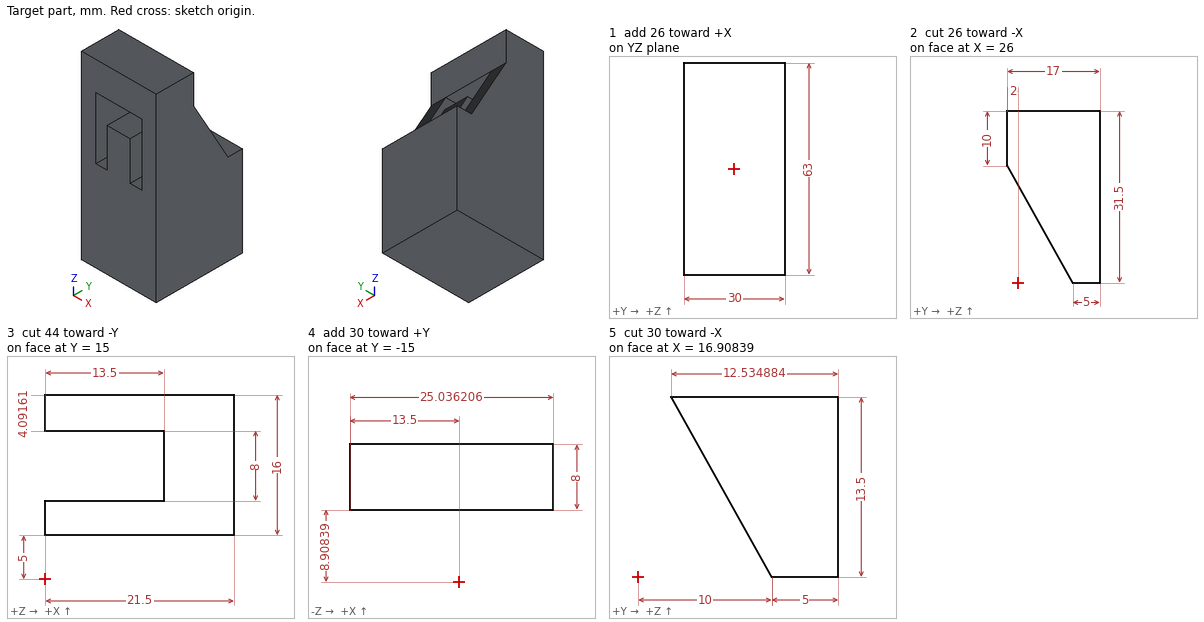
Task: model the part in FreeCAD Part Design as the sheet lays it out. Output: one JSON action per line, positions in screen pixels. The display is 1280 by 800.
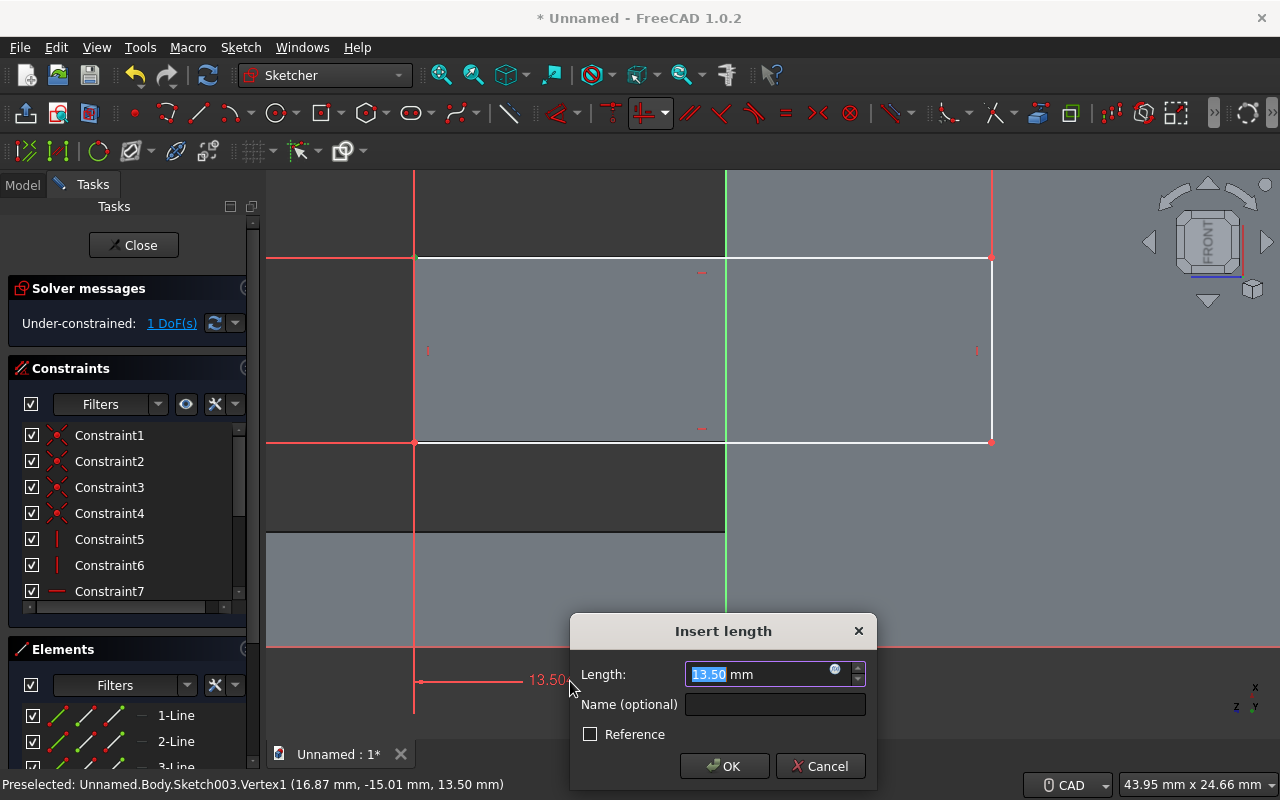
{"action": "type", "text": "13.5"}
{"action": "key", "text": "Return"}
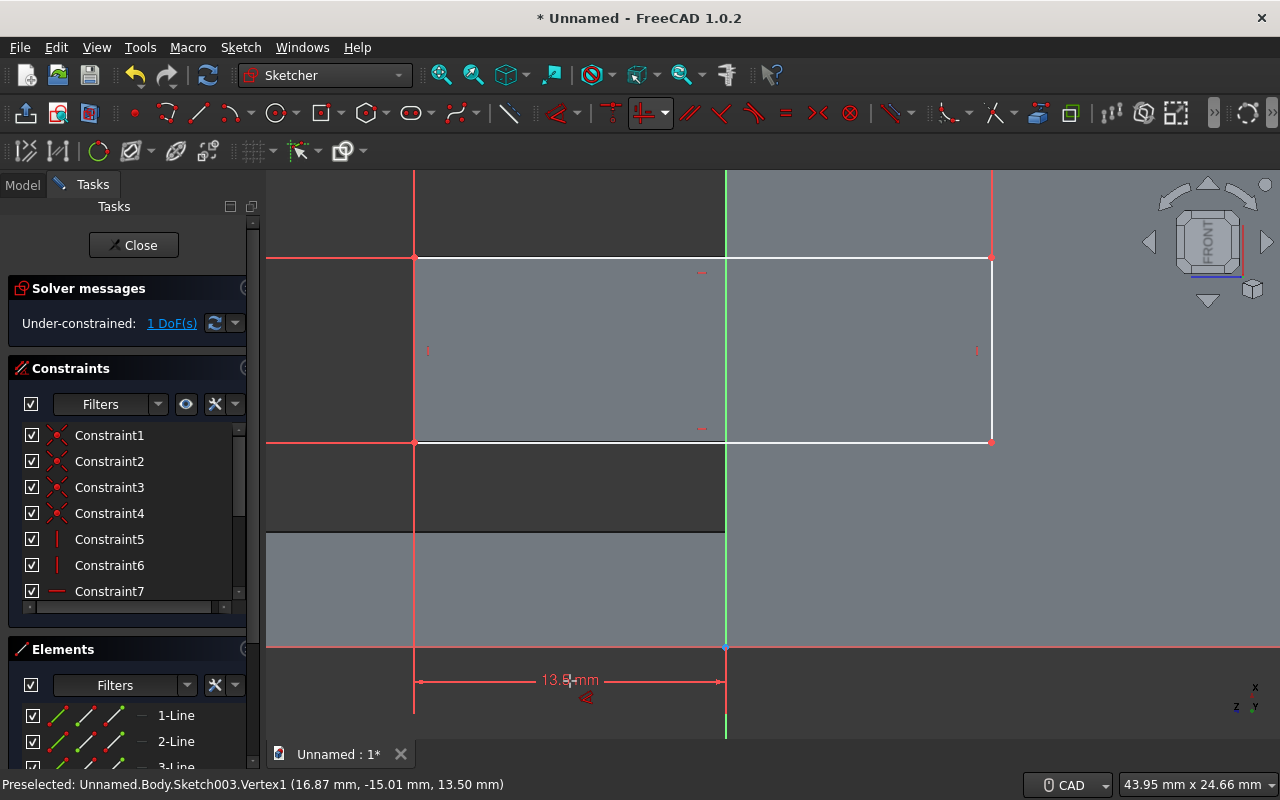
{"action": "left_click", "coordinate": [414, 443]}
{"action": "left_click", "coordinate": [380, 545]}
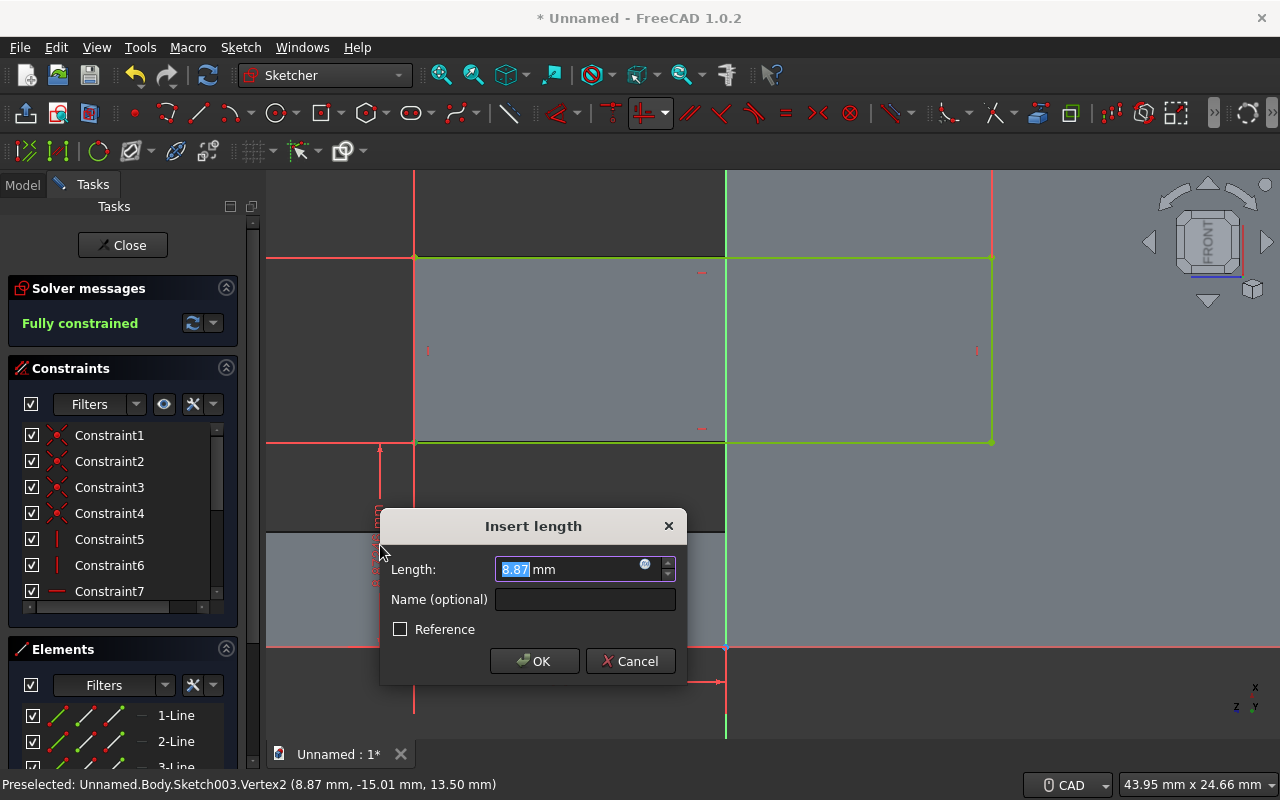
{"action": "type", "text": "8.90839"}
{"action": "key", "text": "Return"}
{"action": "key", "text": "Escape"}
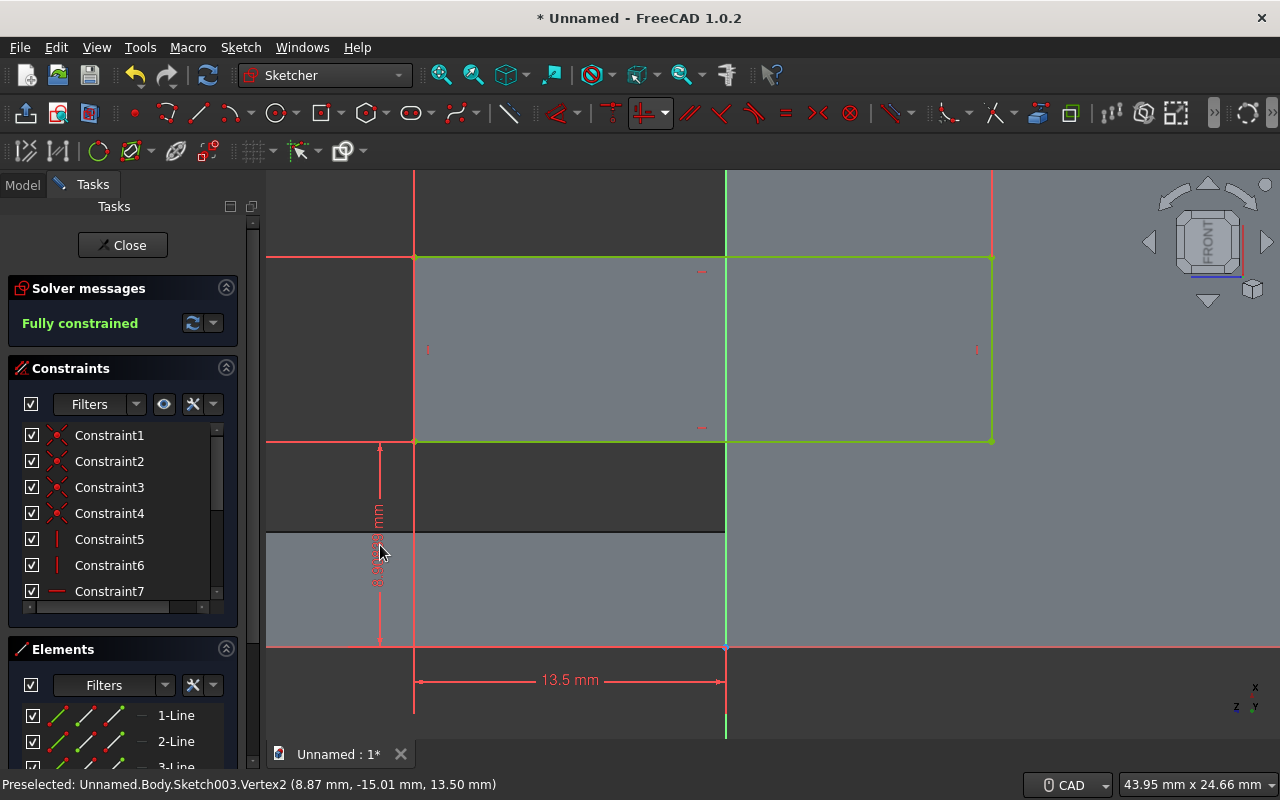
{"action": "left_click", "coordinate": [123, 245]}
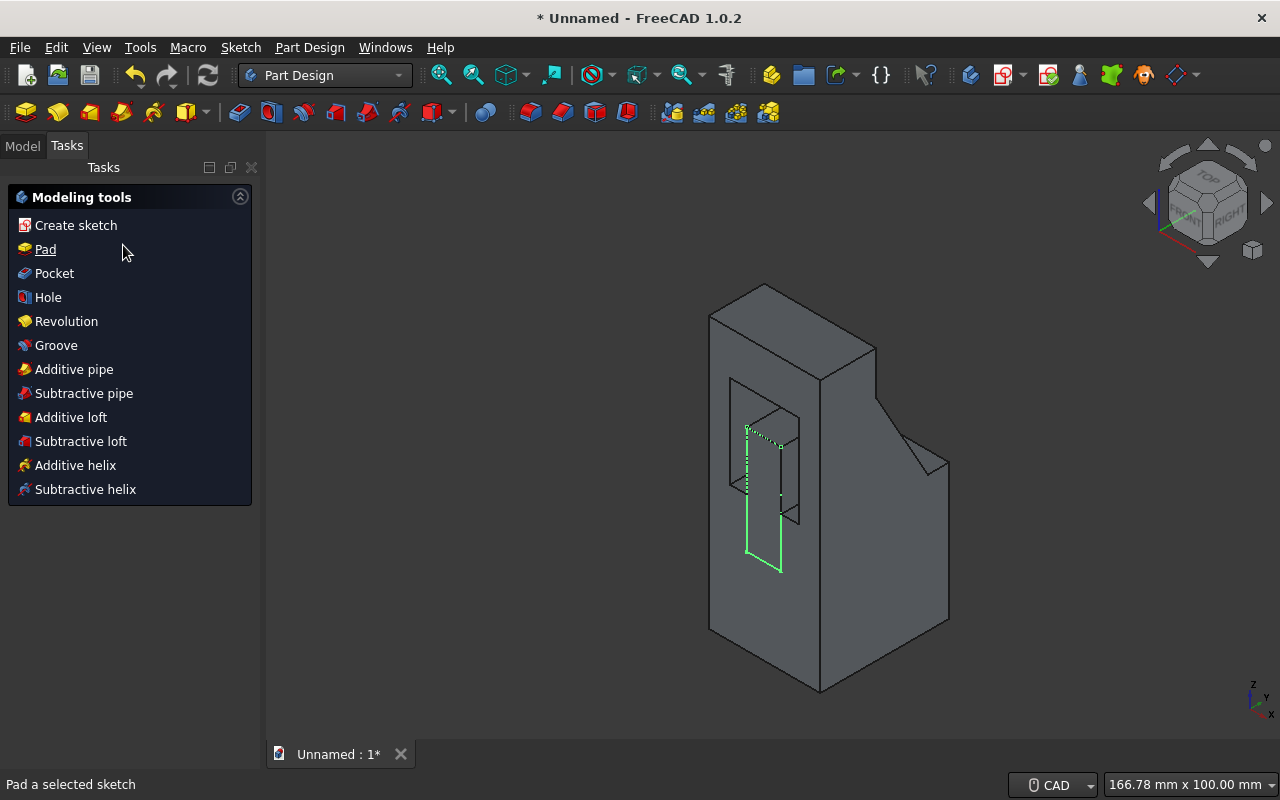
{"action": "left_click", "coordinate": [26, 112]}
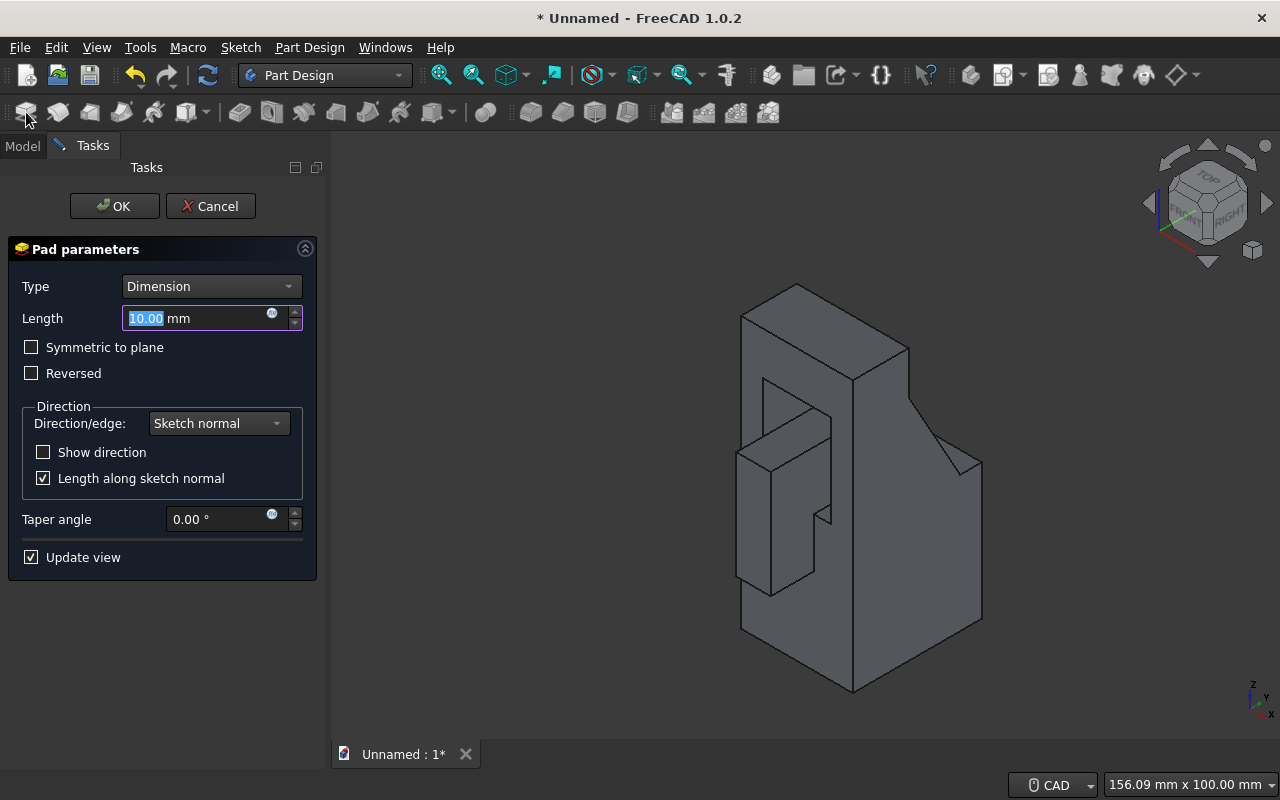
{"action": "type", "text": "30"}
{"action": "key", "text": "Tab"}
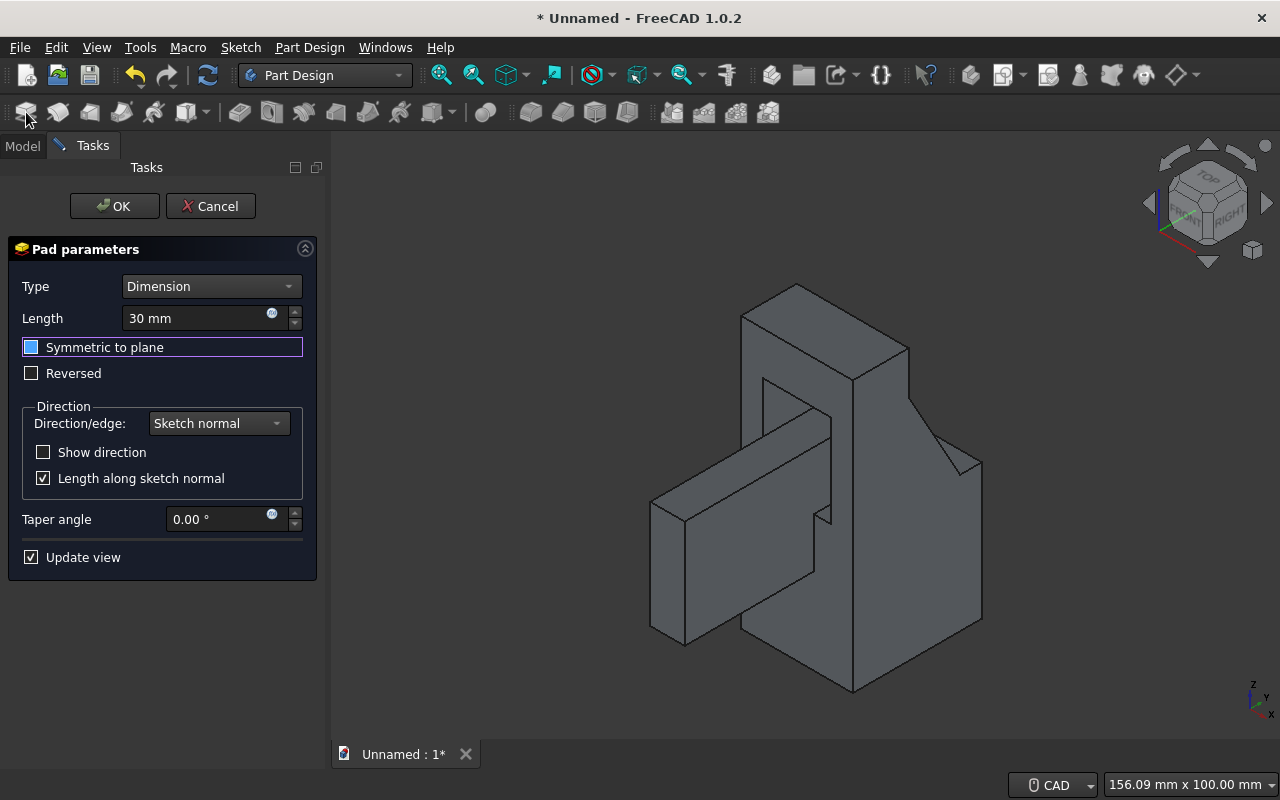
{"action": "left_click", "coordinate": [30, 373]}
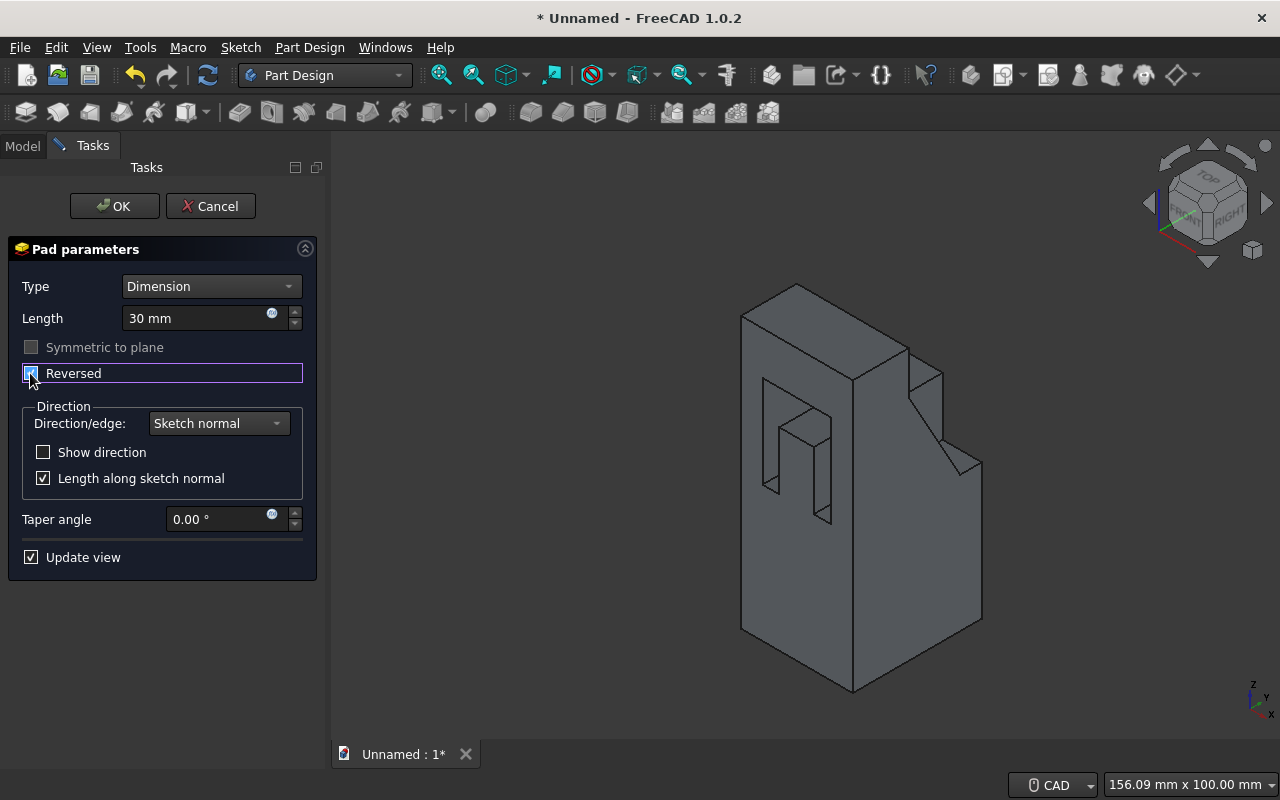
{"action": "left_click", "coordinate": [115, 206]}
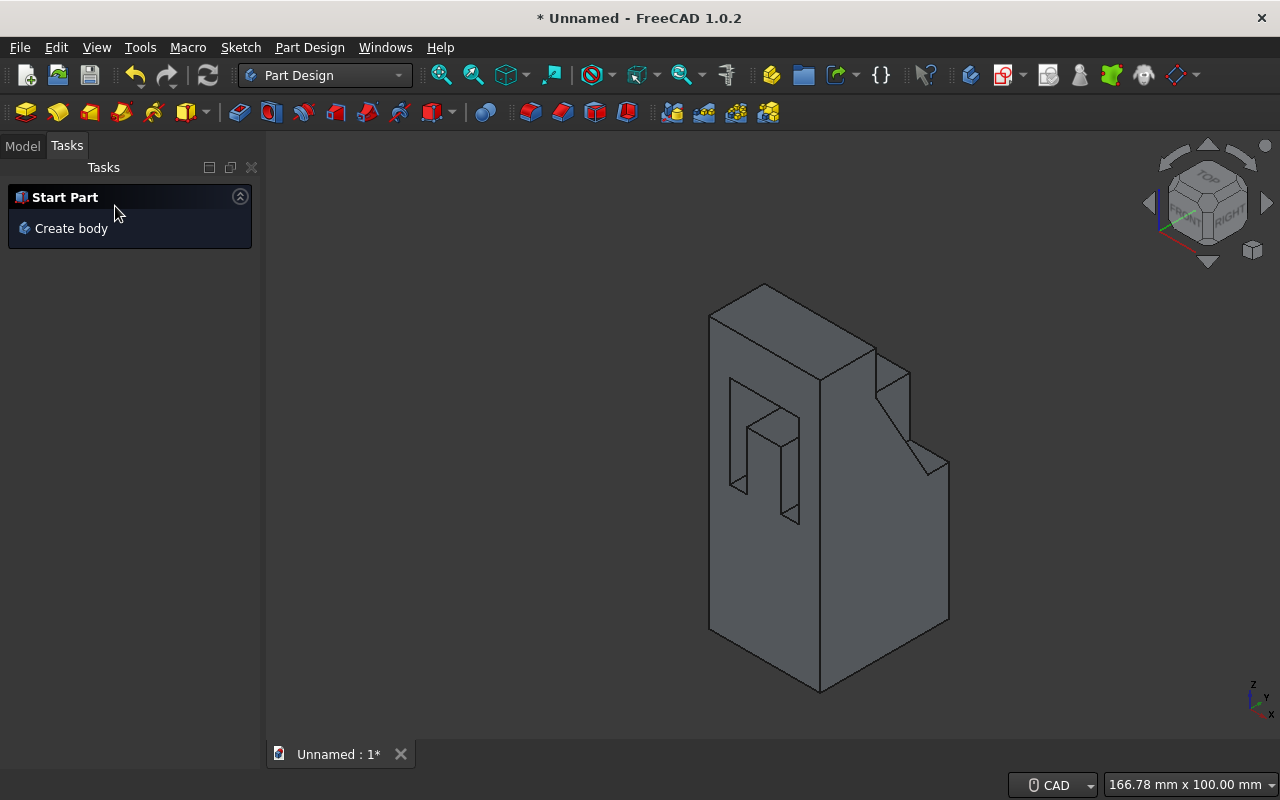
{"action": "key", "text": "3"}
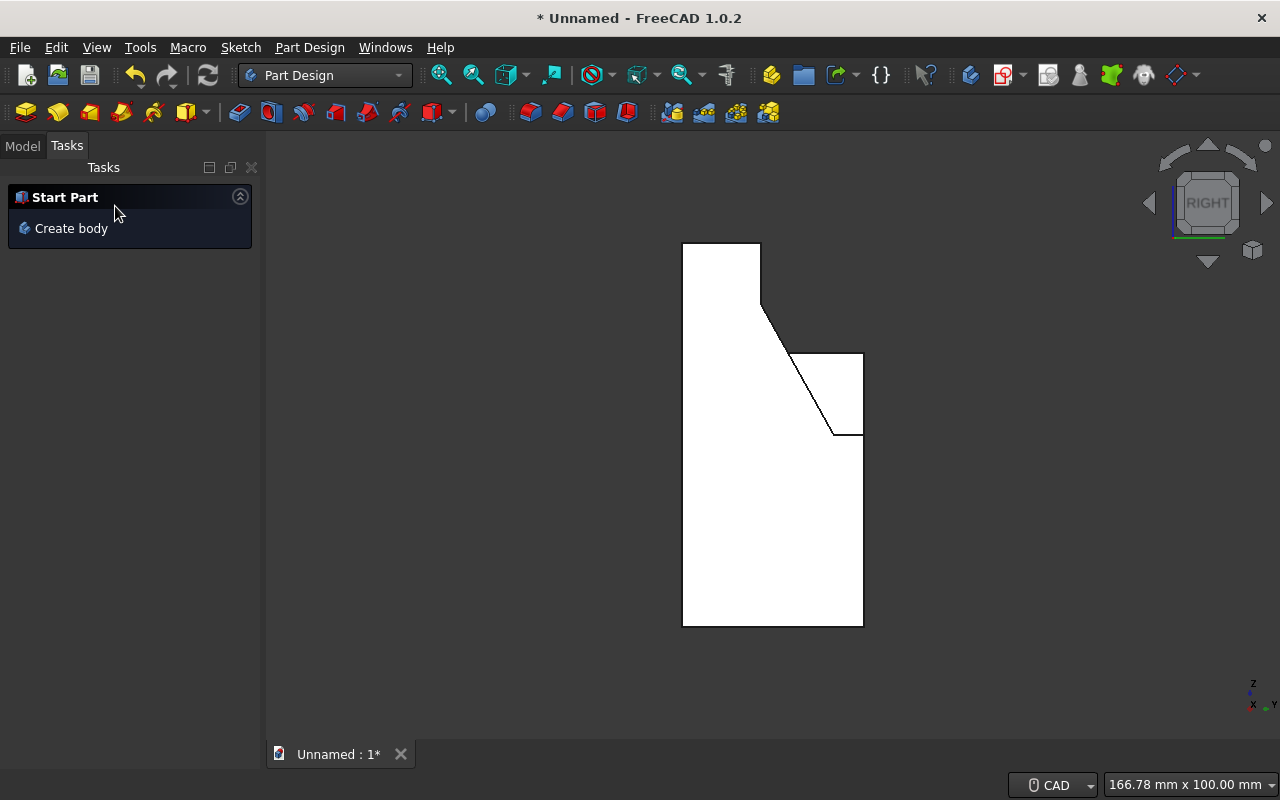
{"action": "left_click", "coordinate": [825, 393]}